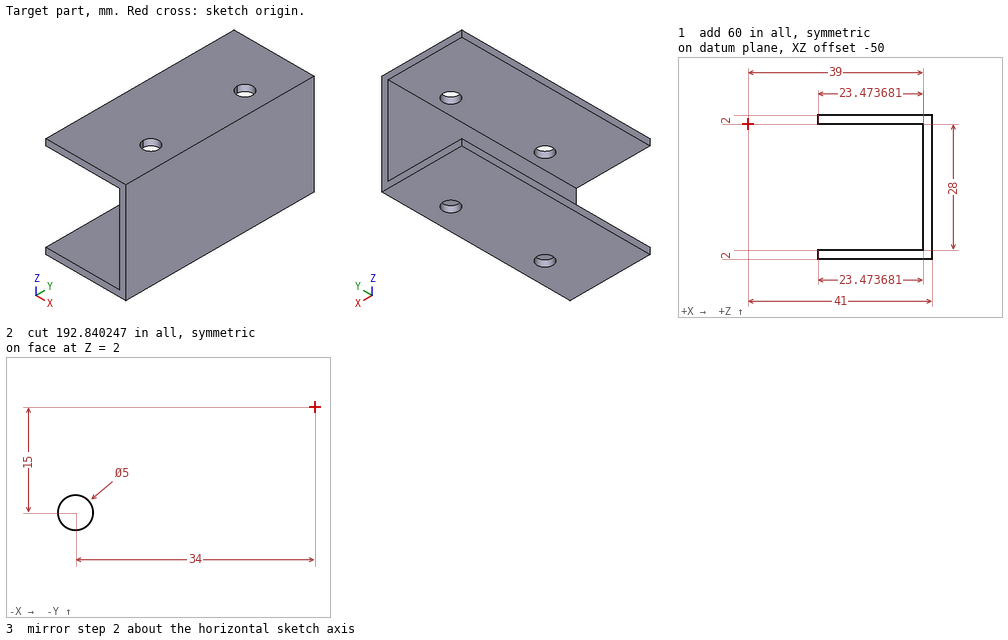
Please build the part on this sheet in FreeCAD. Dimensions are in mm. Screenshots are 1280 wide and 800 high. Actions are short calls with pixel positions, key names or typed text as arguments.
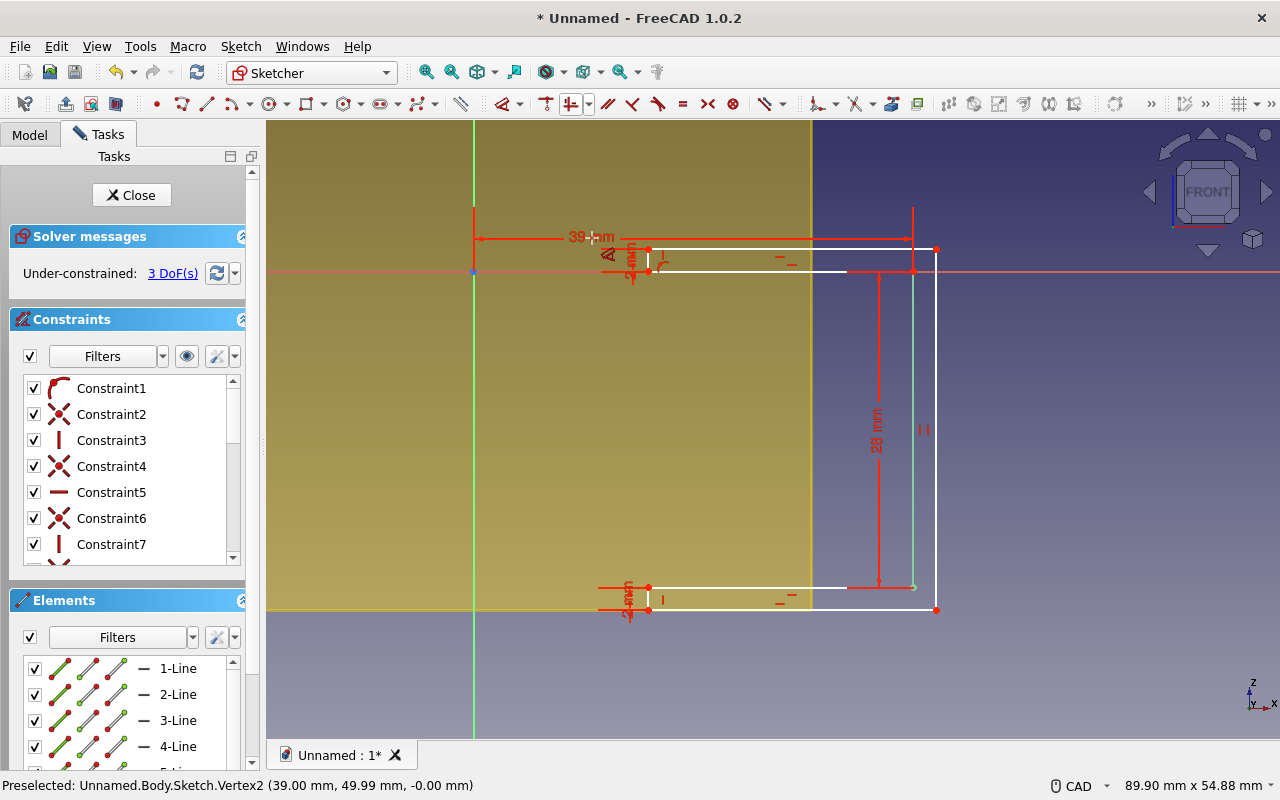
click(936, 610)
click(705, 644)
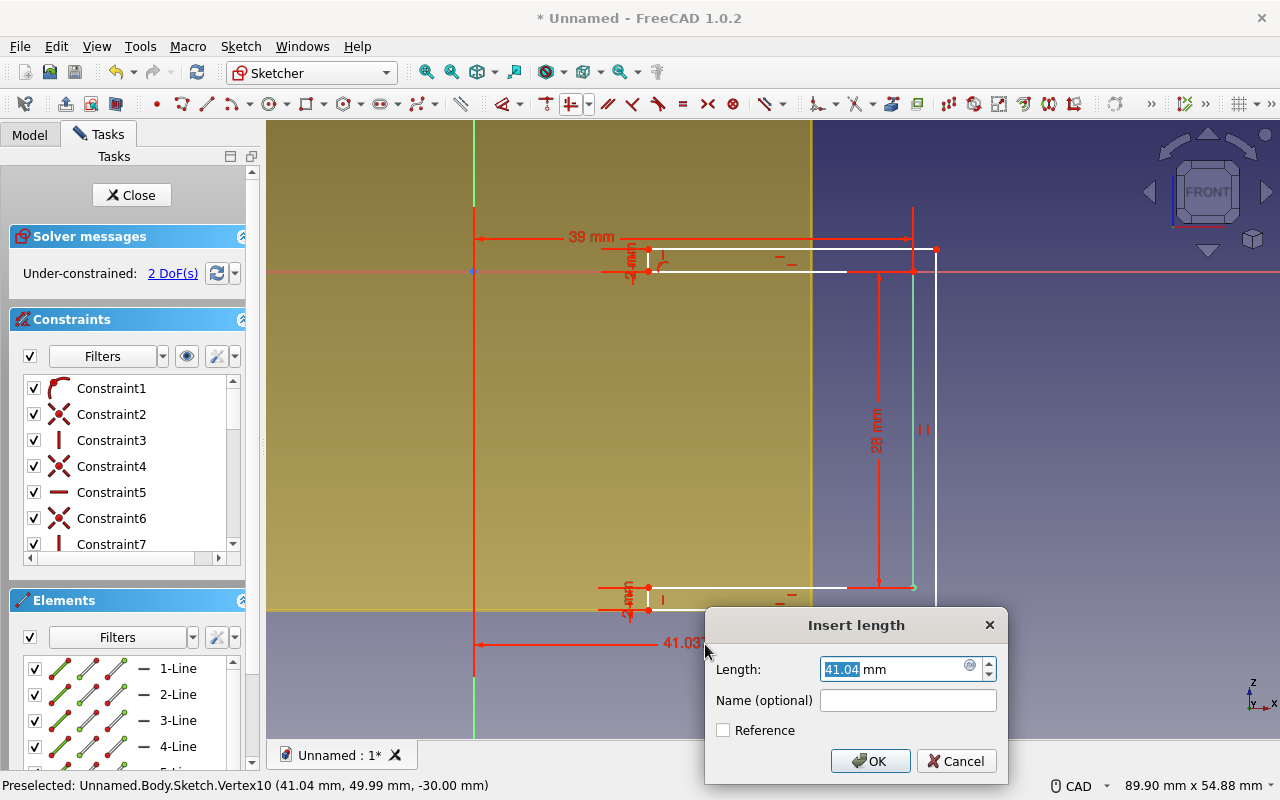
text(41)
key(Return)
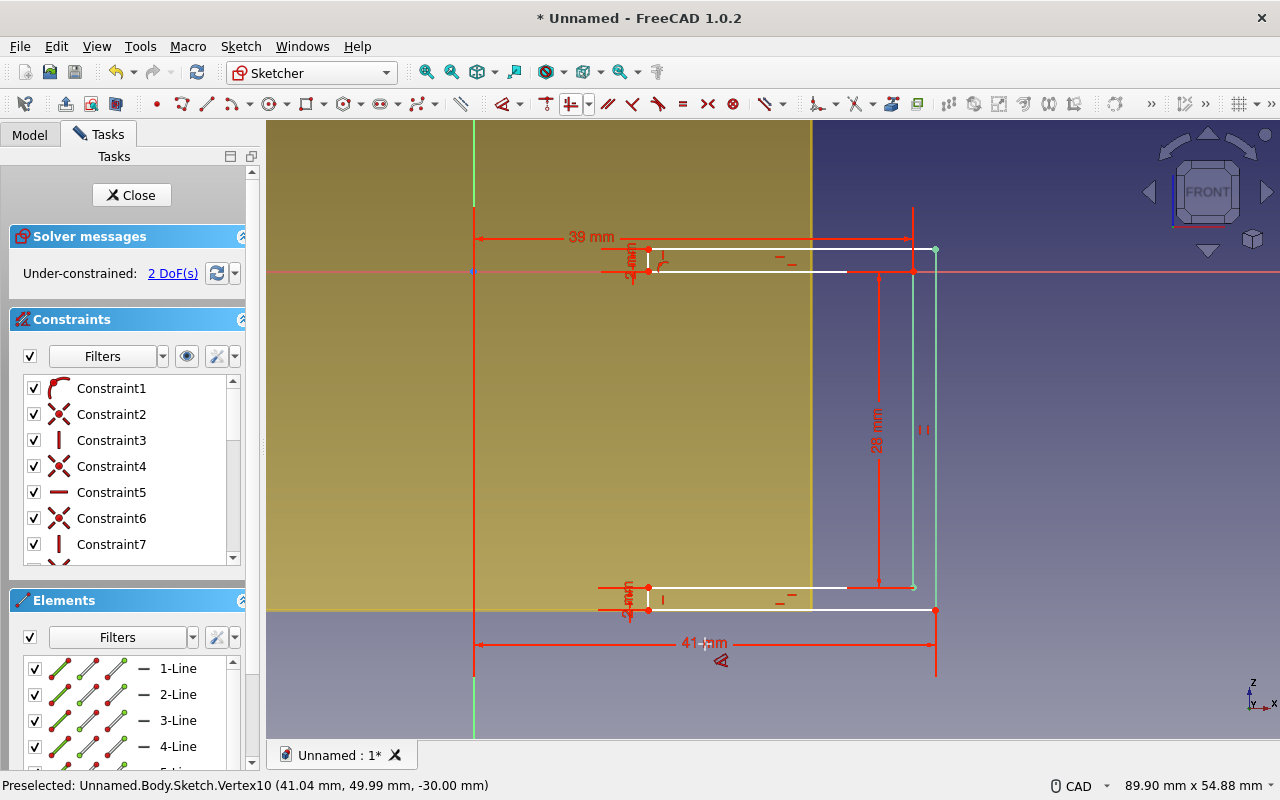
click(728, 272)
click(781, 306)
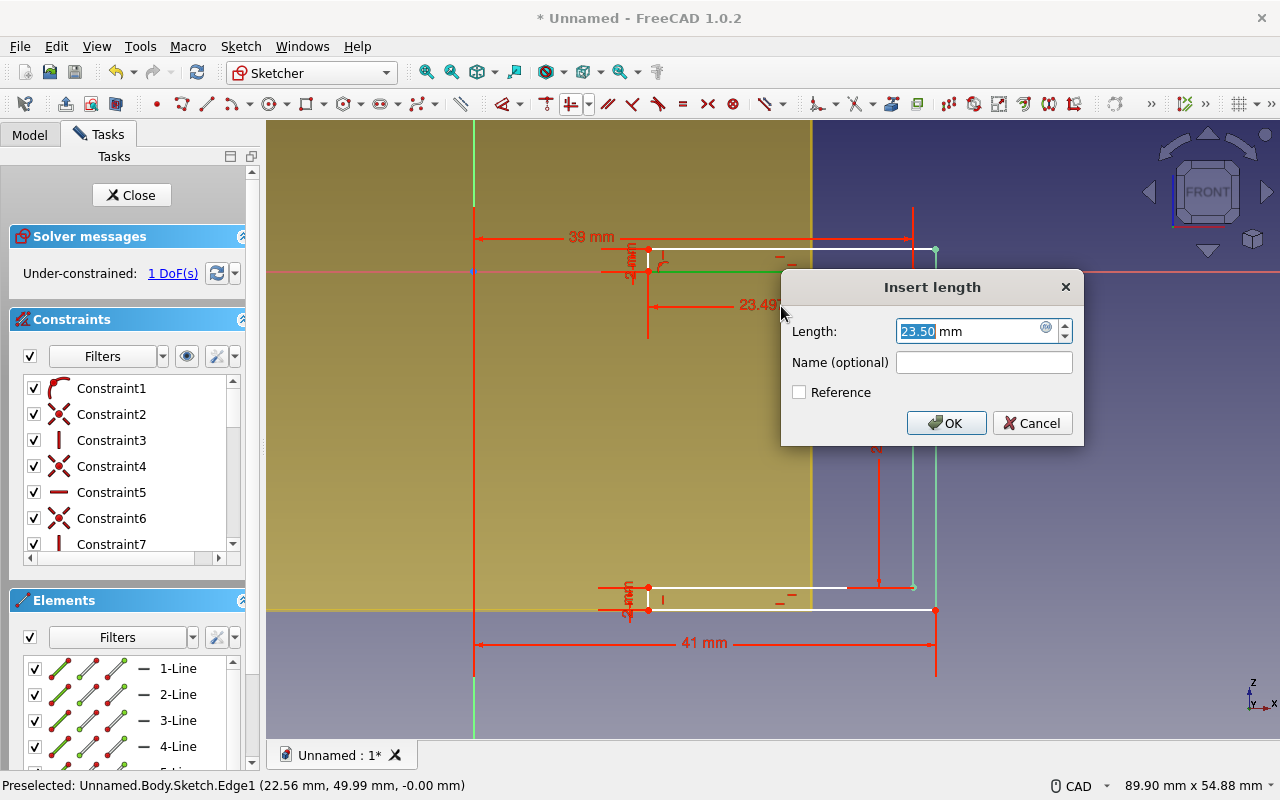
text(23.473681)
key(Return)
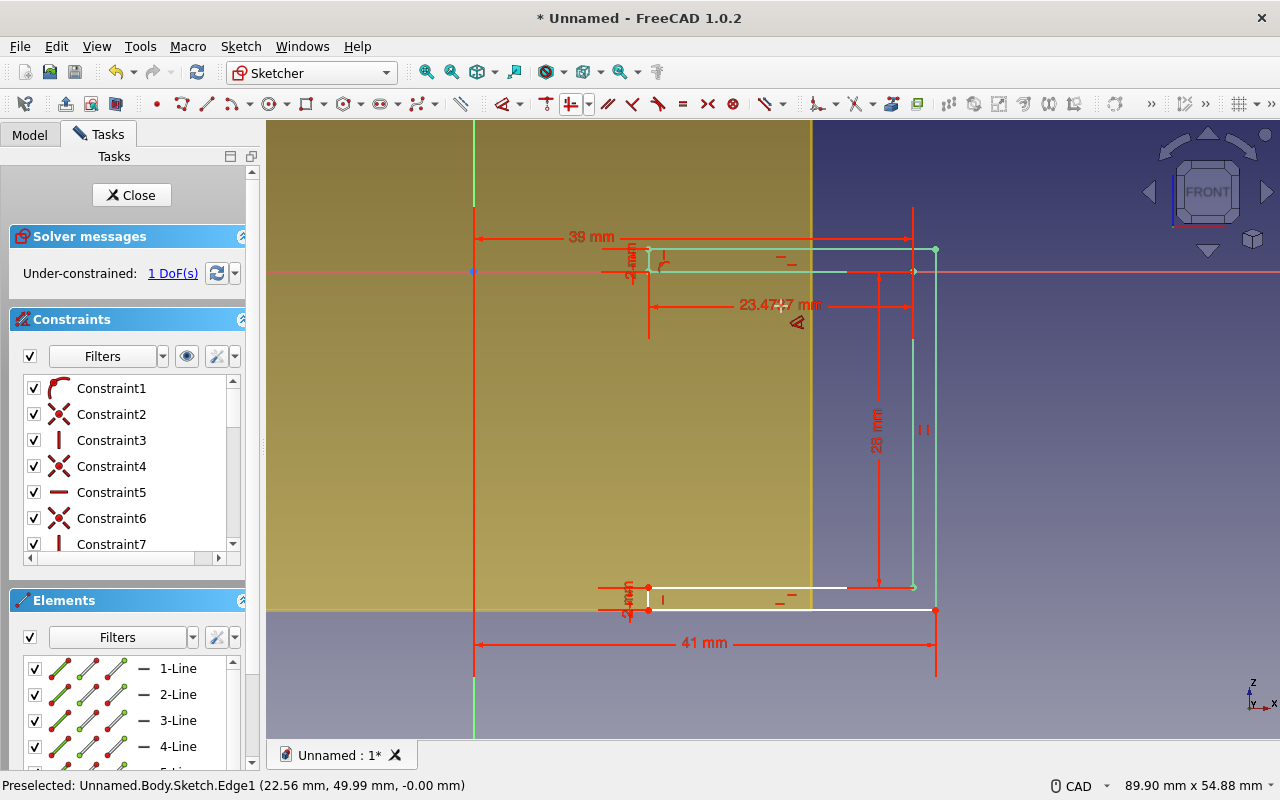
click(834, 588)
click(781, 554)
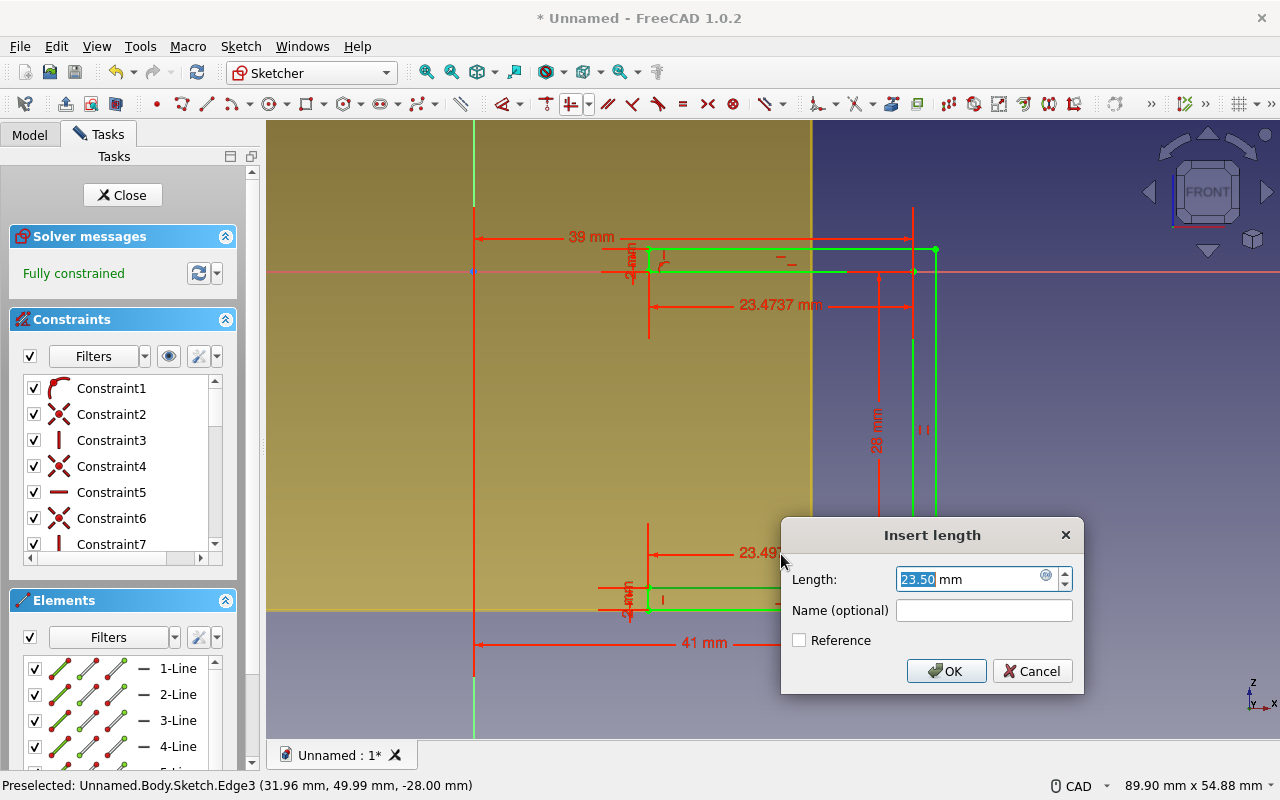
text(23.473681)
key(Return)
key(Escape)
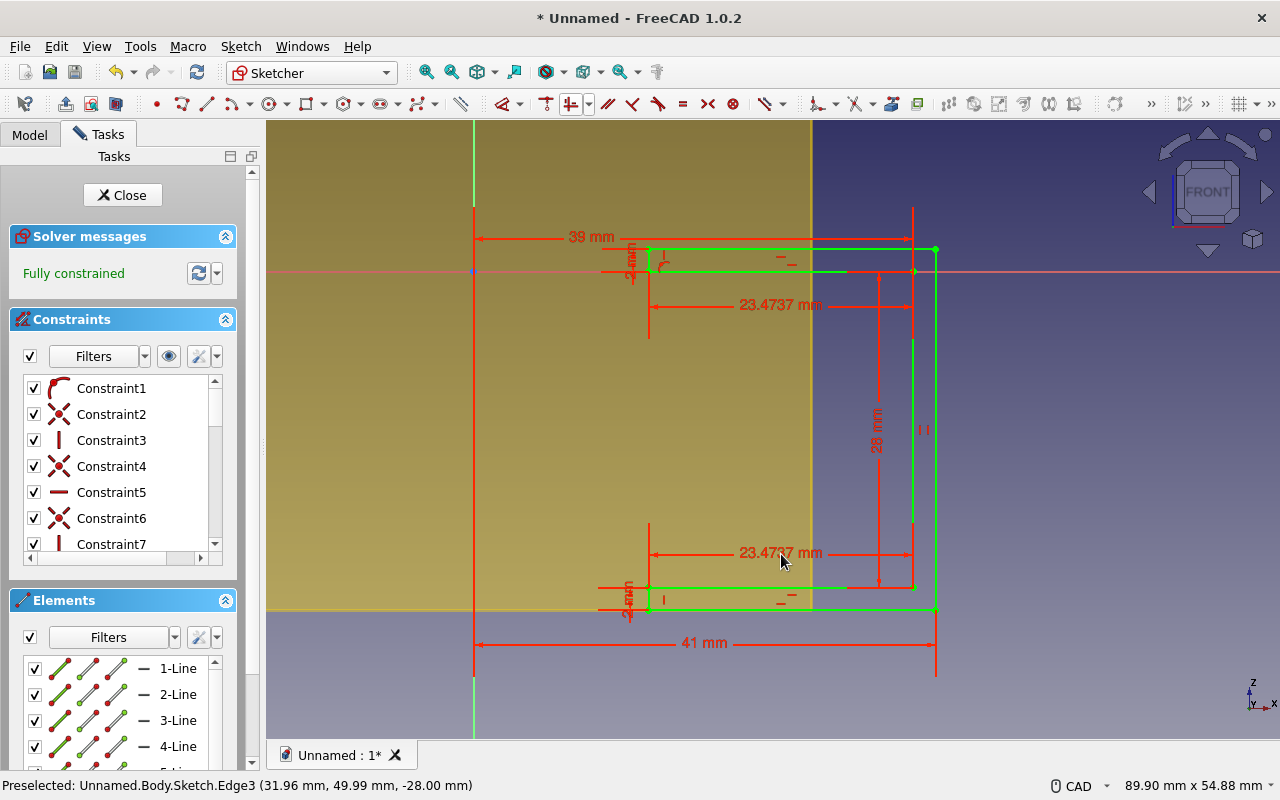
click(123, 195)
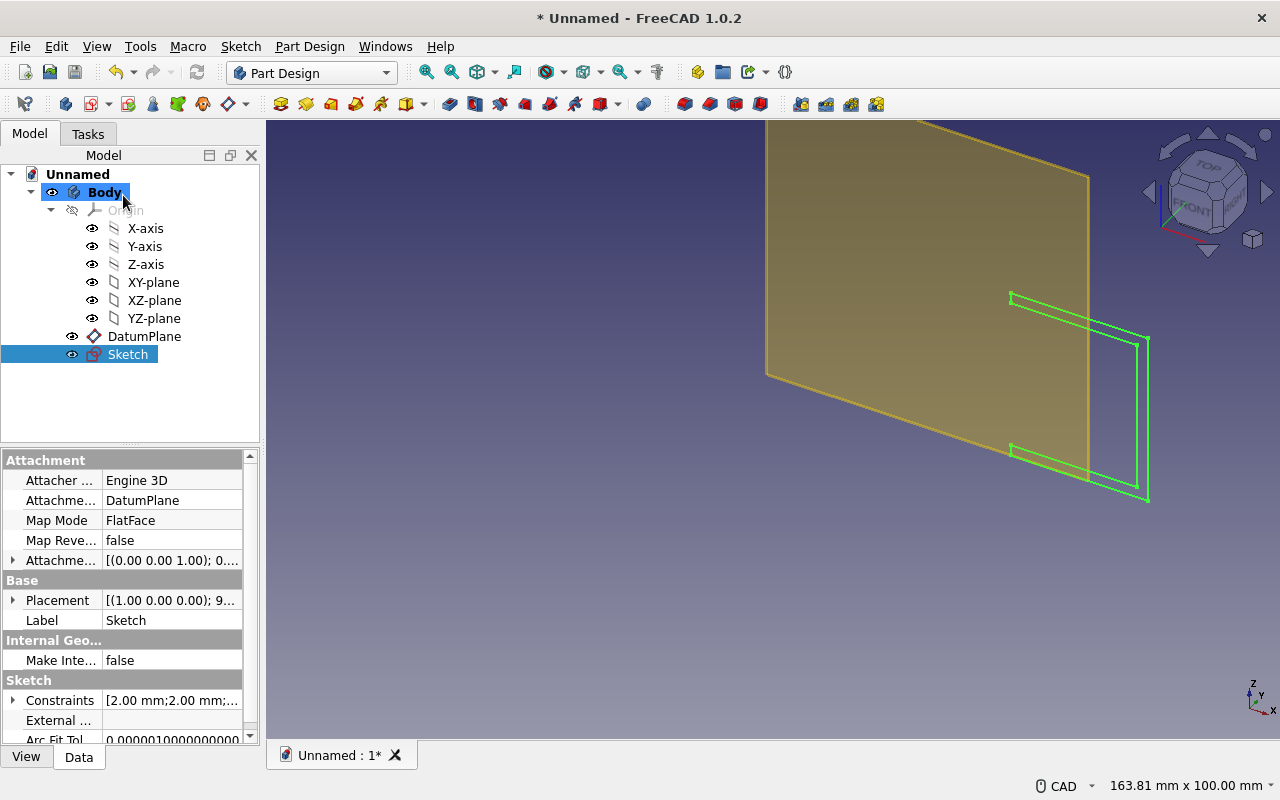
click(281, 104)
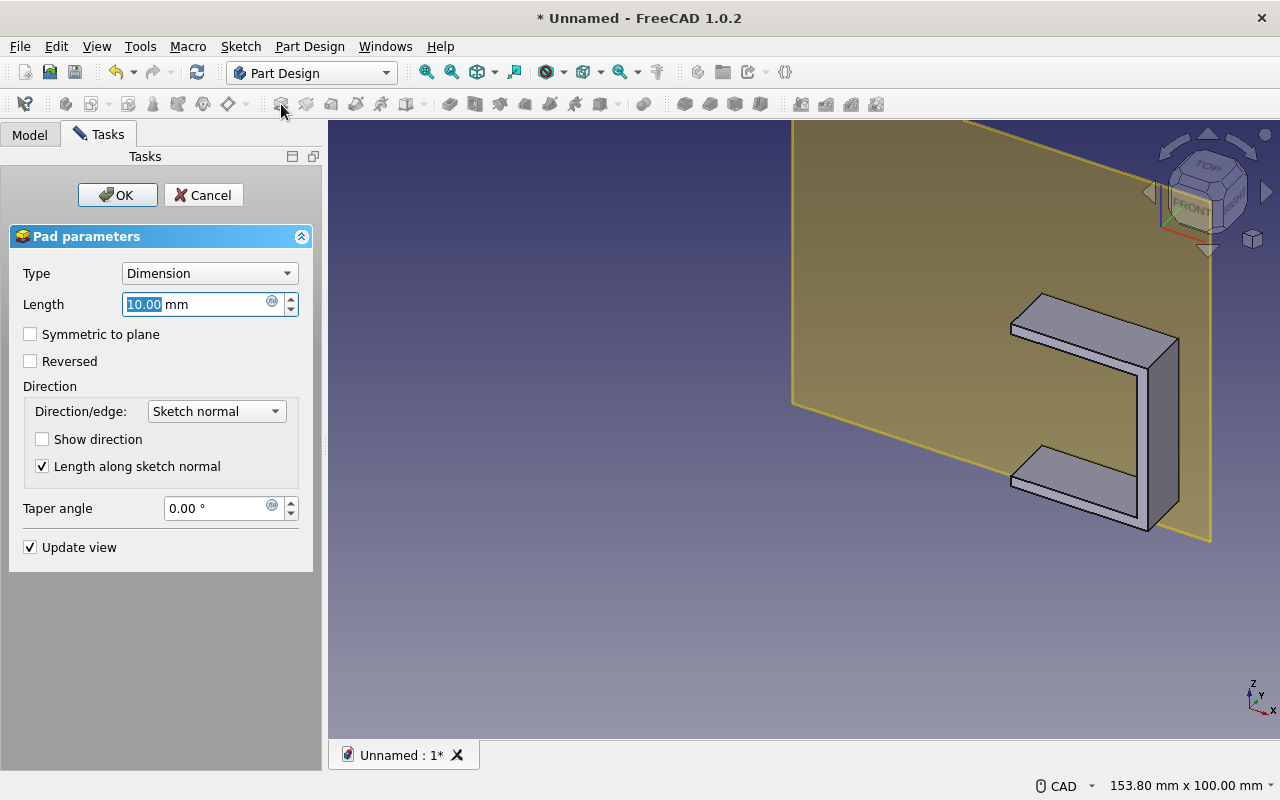
text(60)
key(Tab)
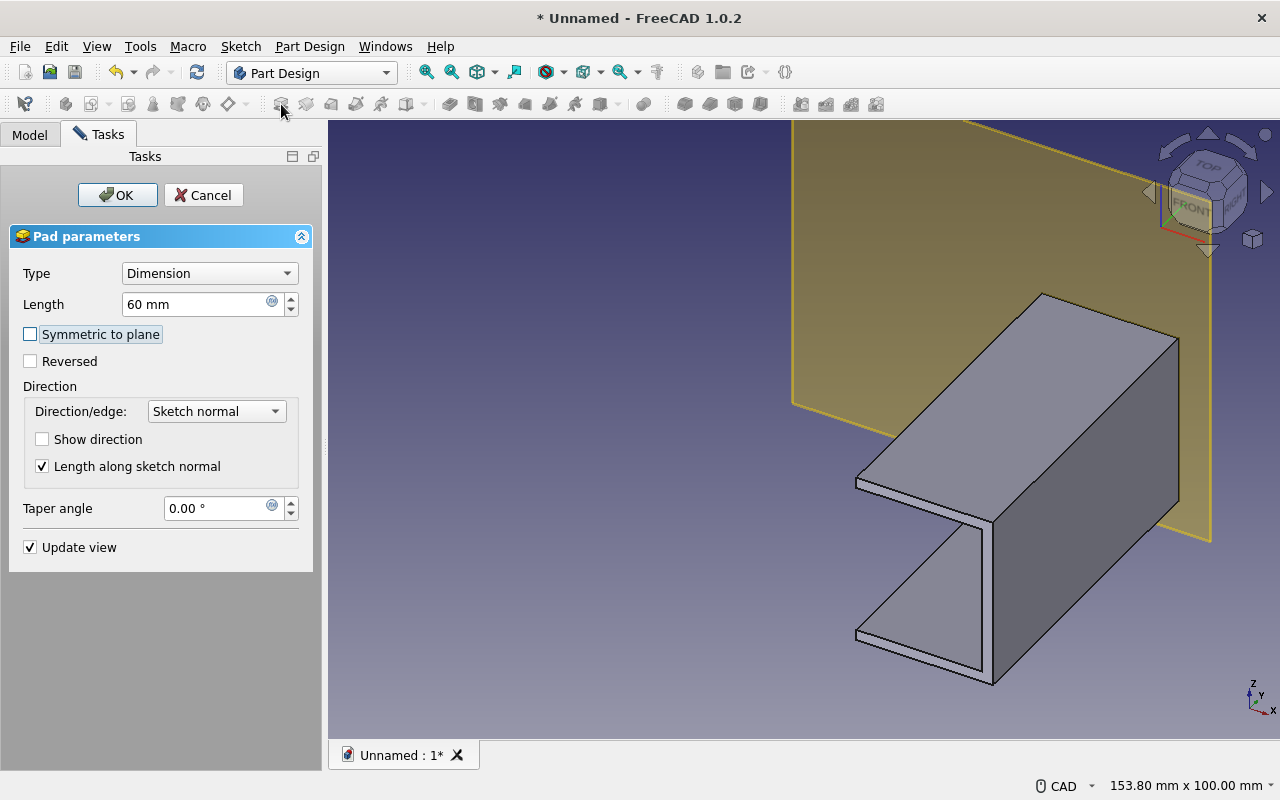
click(31, 334)